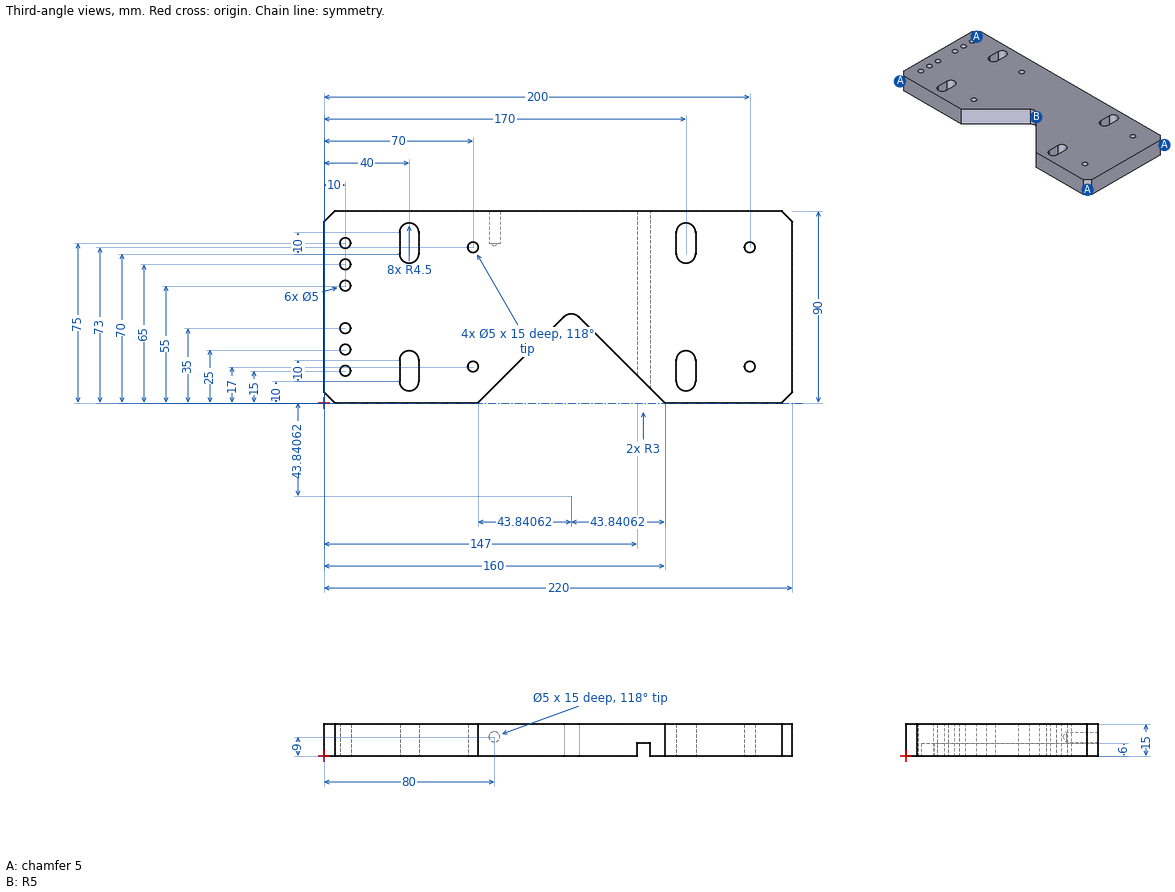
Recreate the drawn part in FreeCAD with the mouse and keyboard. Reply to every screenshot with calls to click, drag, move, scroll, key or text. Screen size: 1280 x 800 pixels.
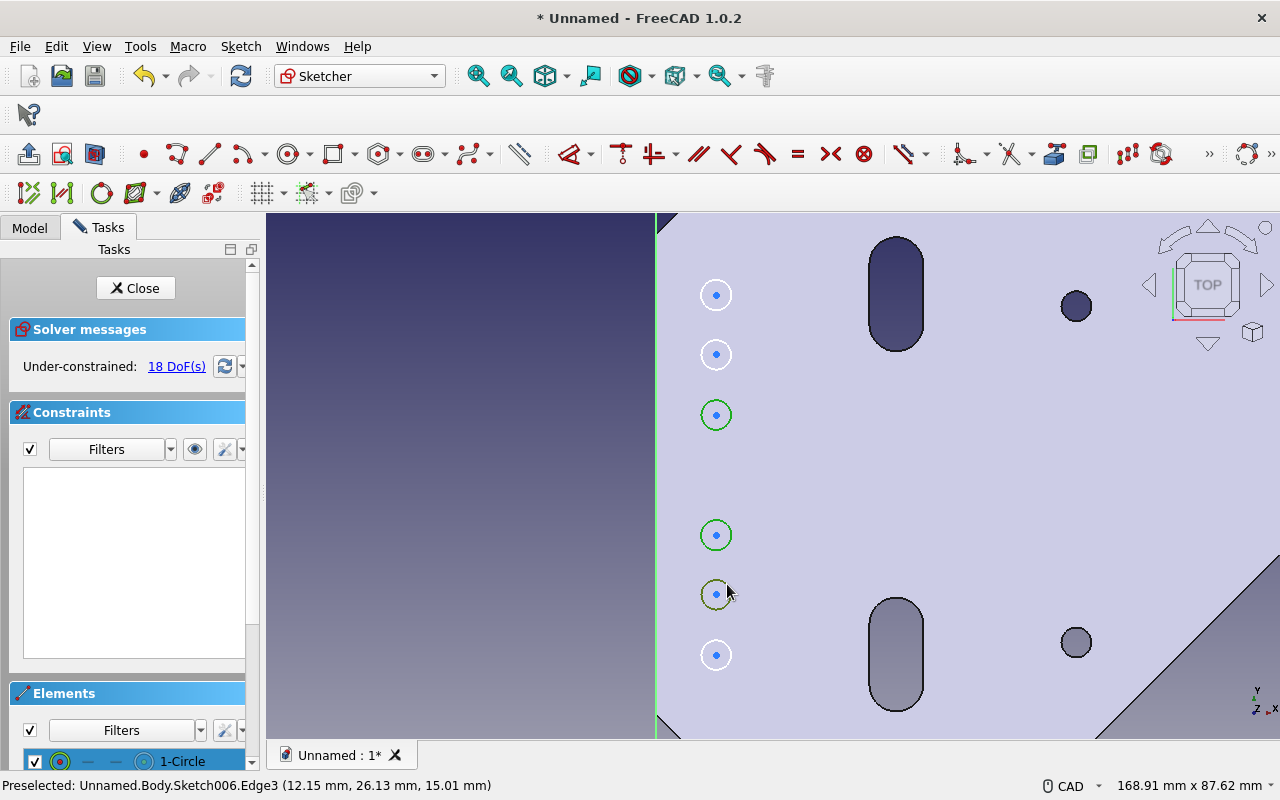
click(727, 344)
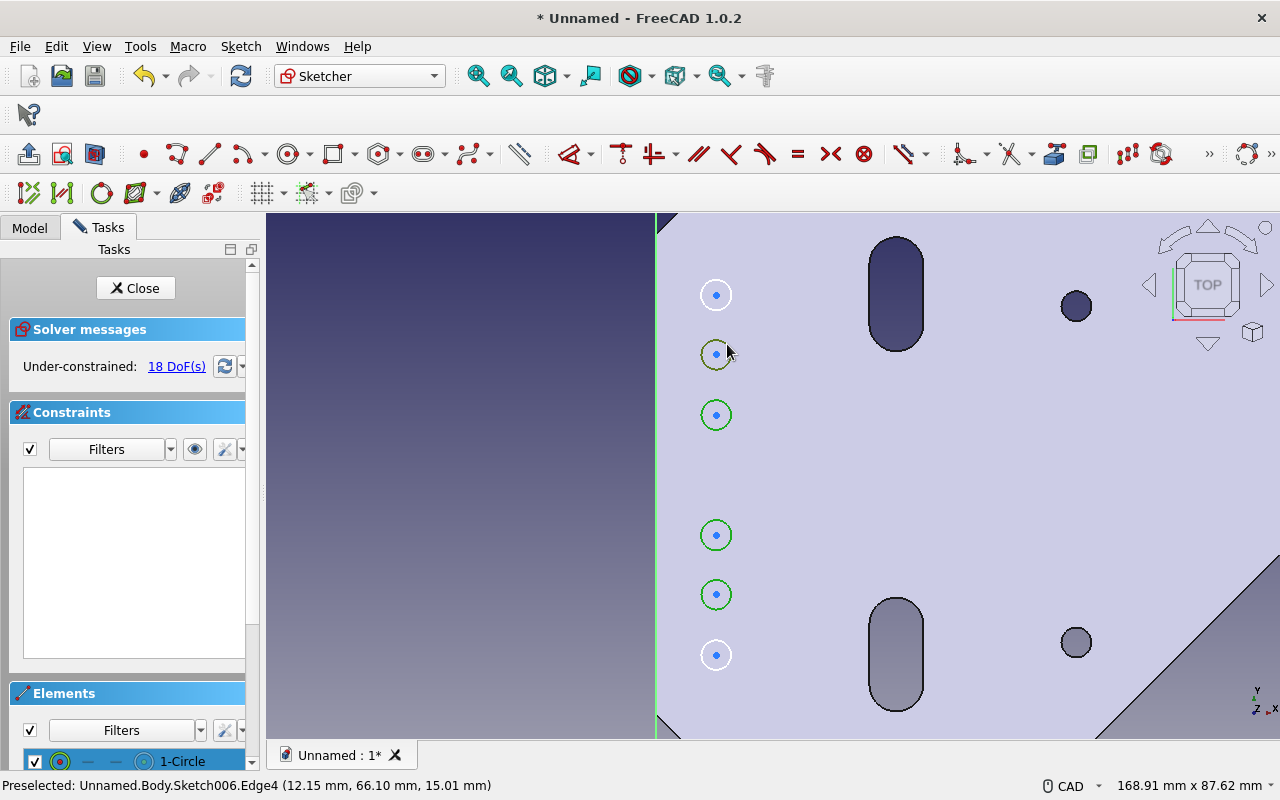
click(727, 284)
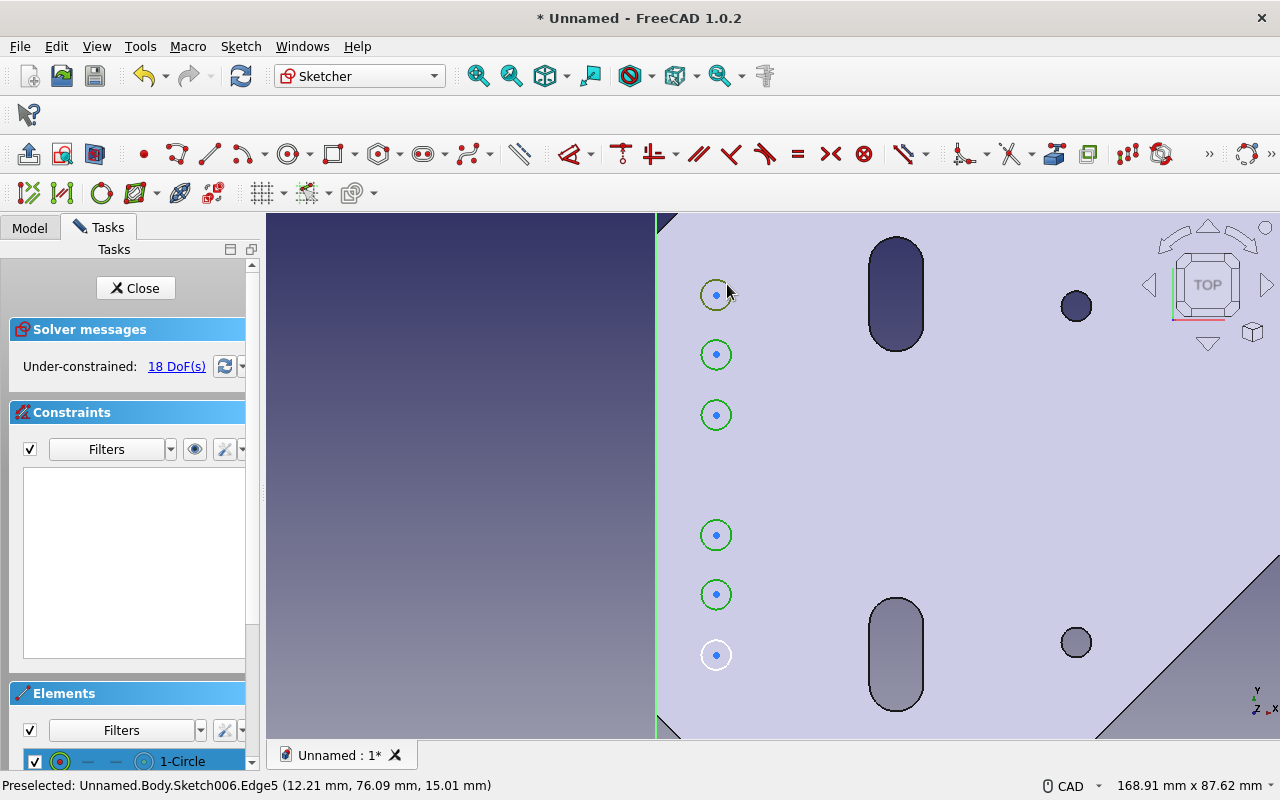
click(727, 645)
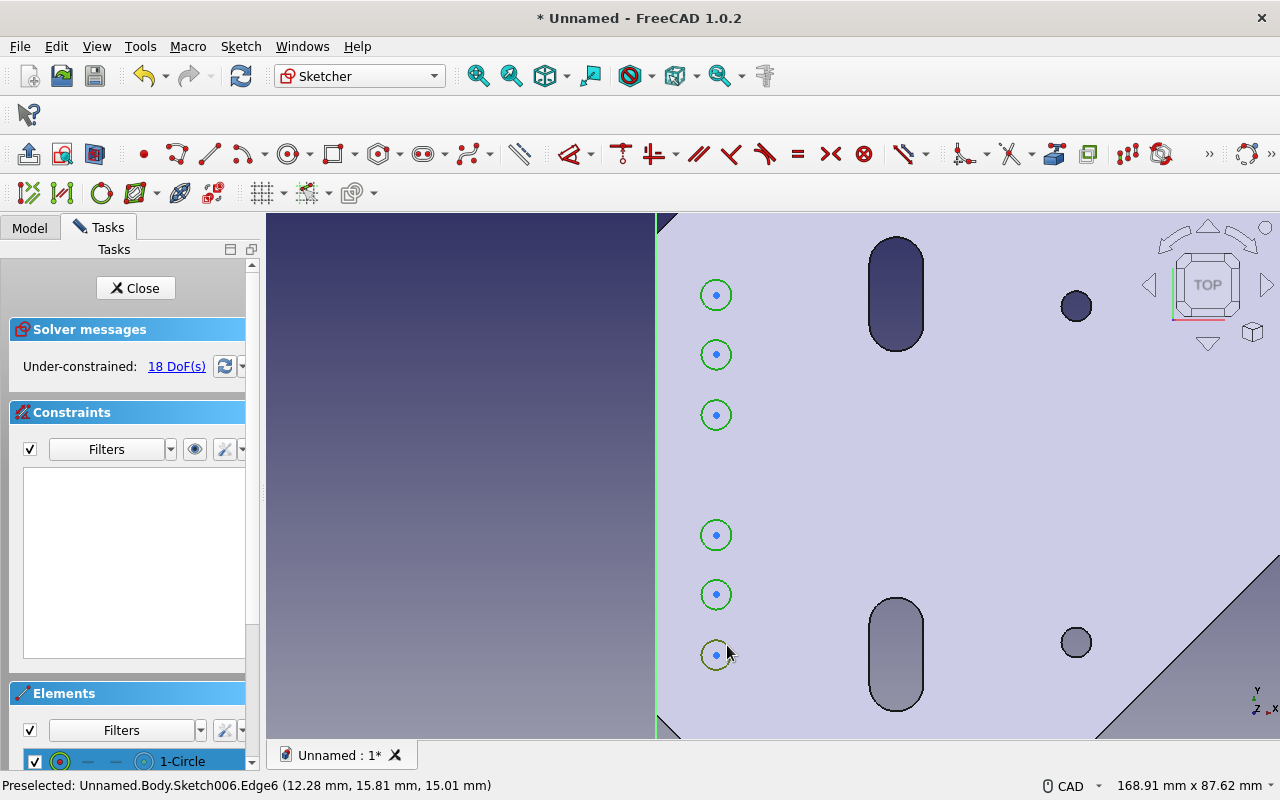
key(e)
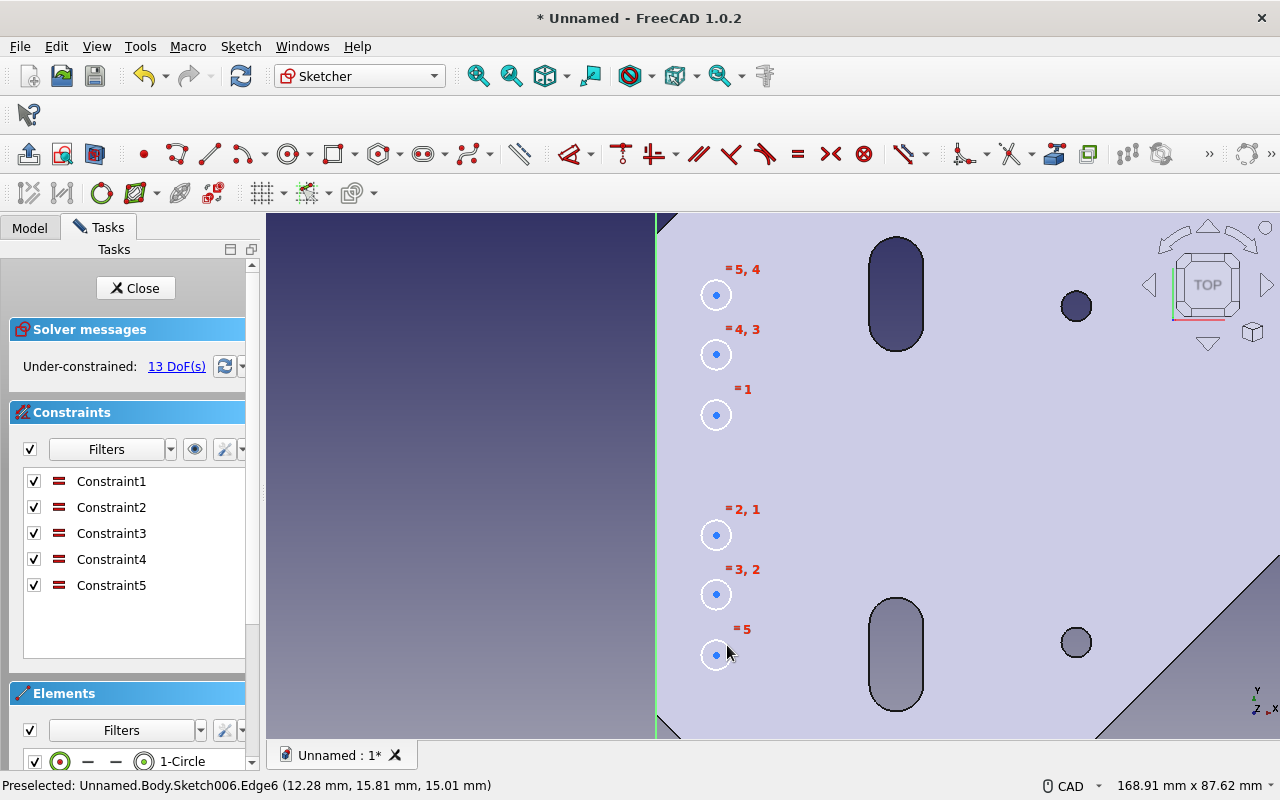
click(568, 154)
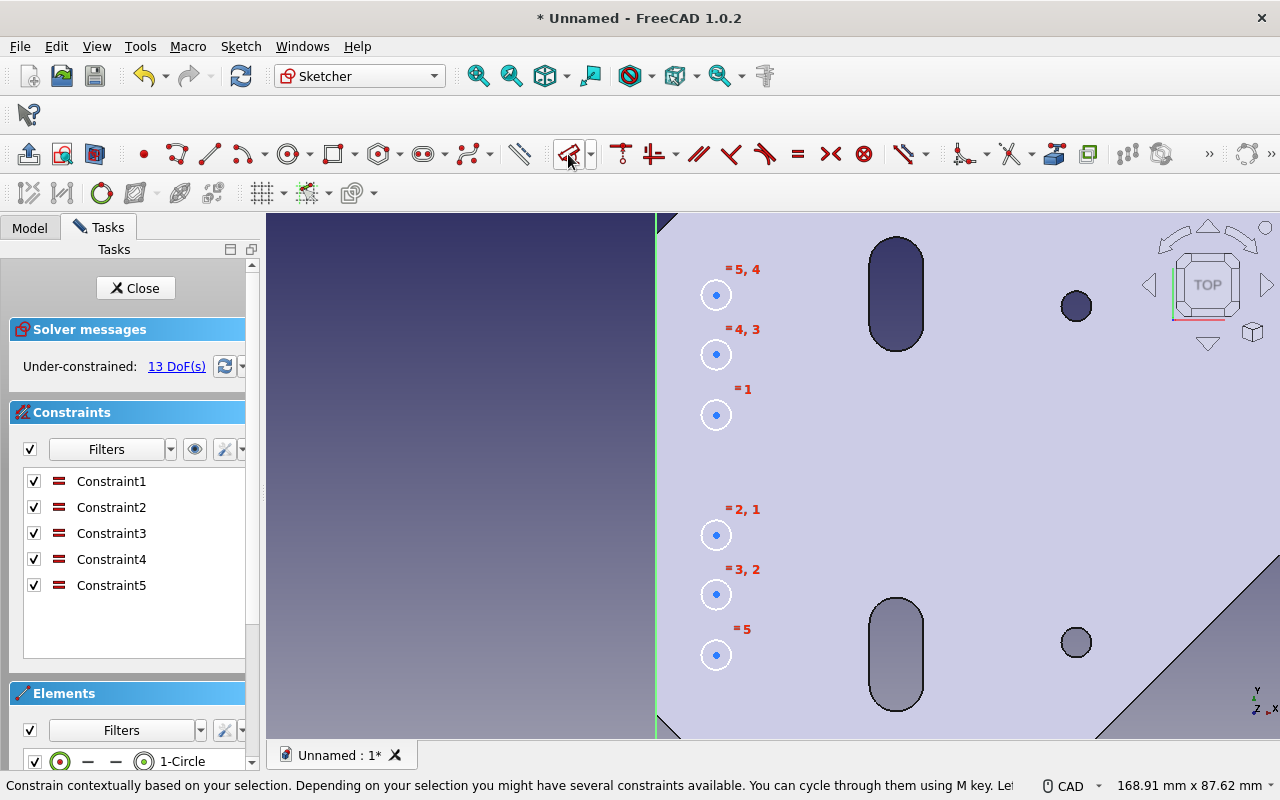
scroll(727, 405, up, 2)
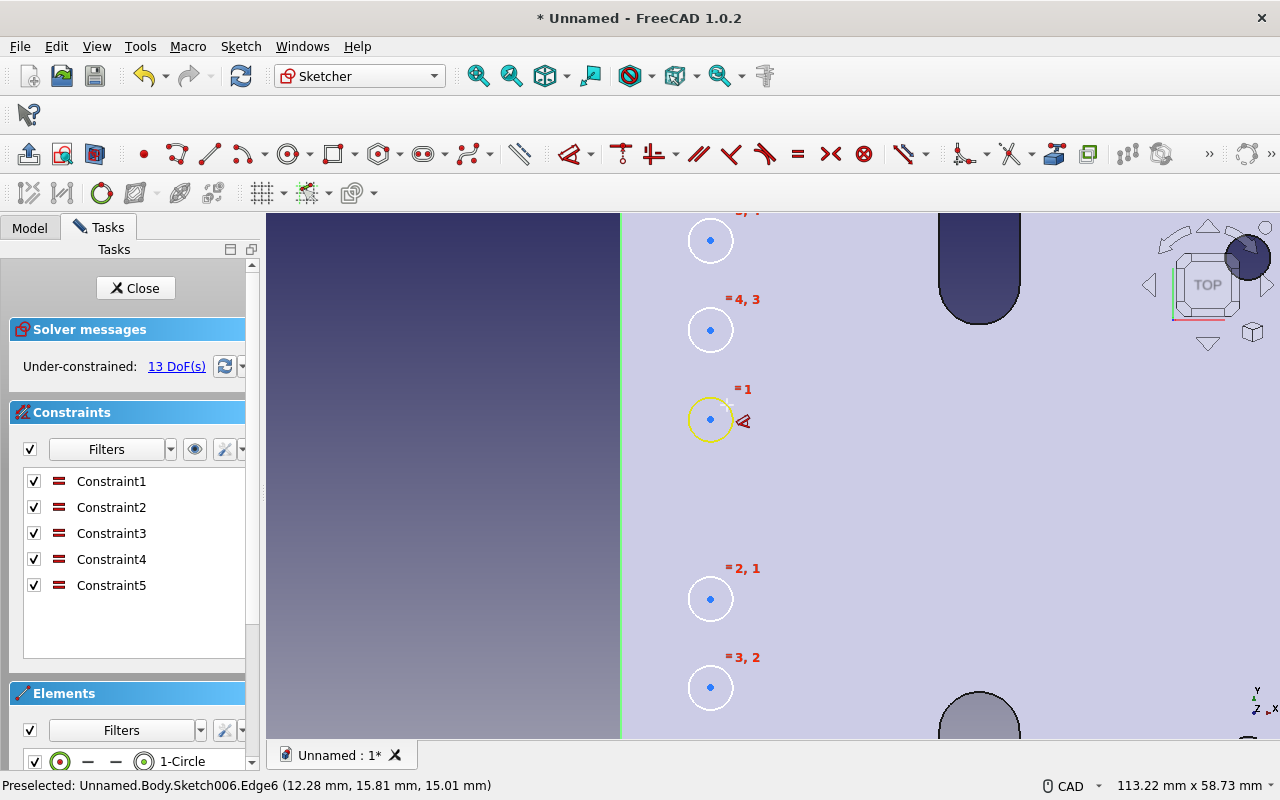
click(726, 404)
click(748, 381)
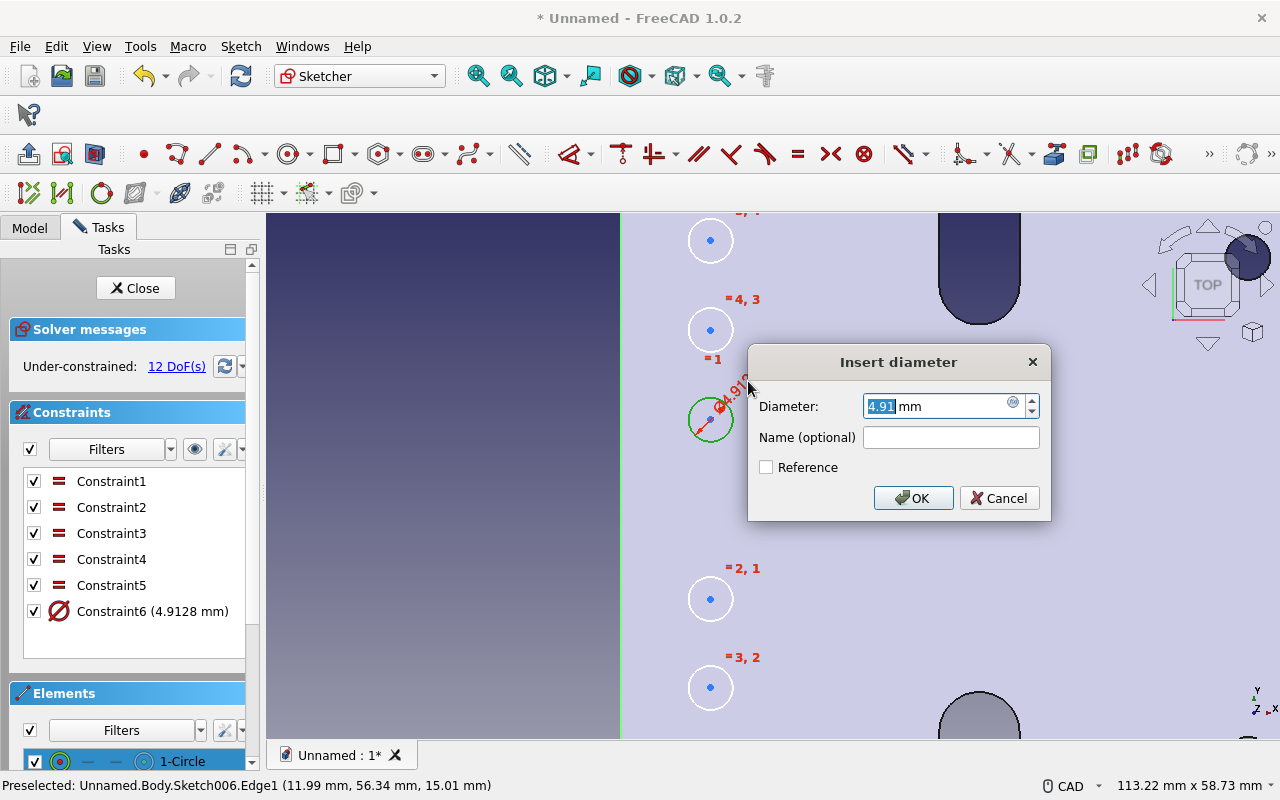
text(5)
key(Return)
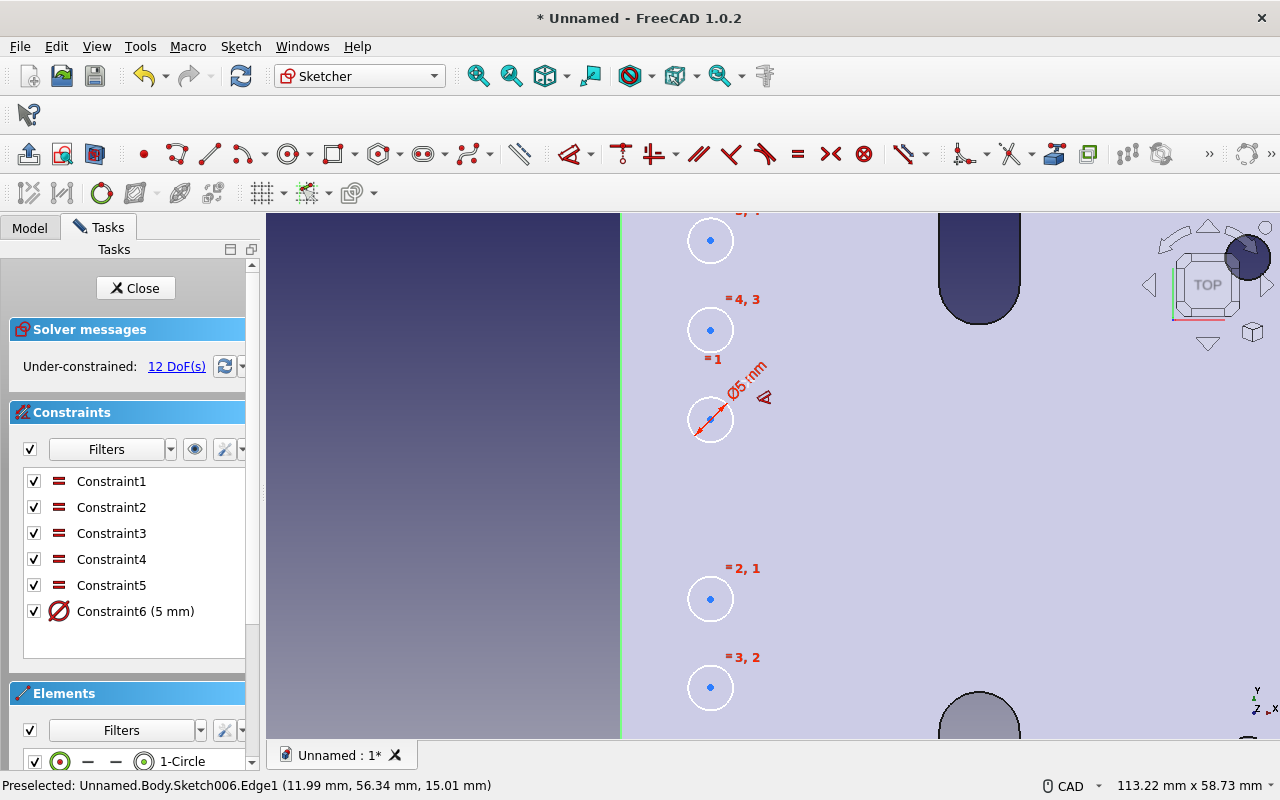
click(711, 420)
click(666, 386)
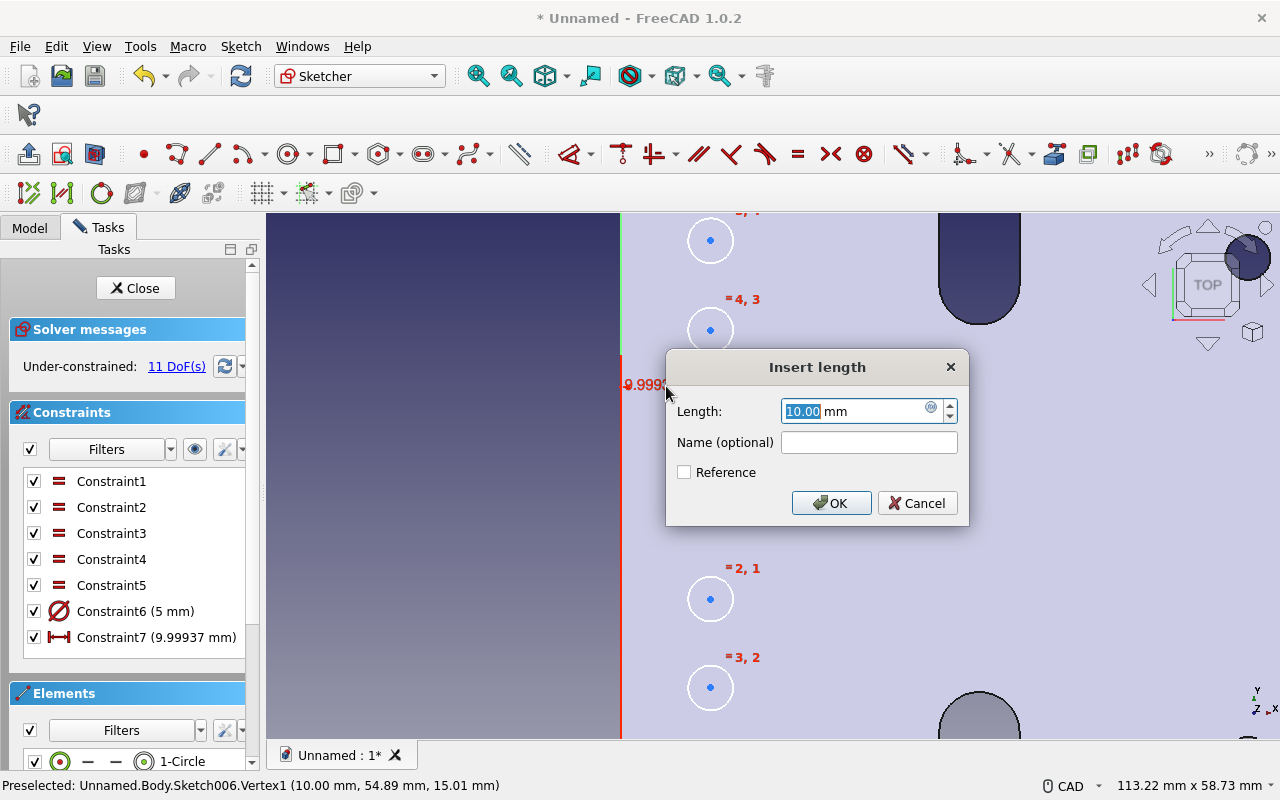
text(10)
key(Return)